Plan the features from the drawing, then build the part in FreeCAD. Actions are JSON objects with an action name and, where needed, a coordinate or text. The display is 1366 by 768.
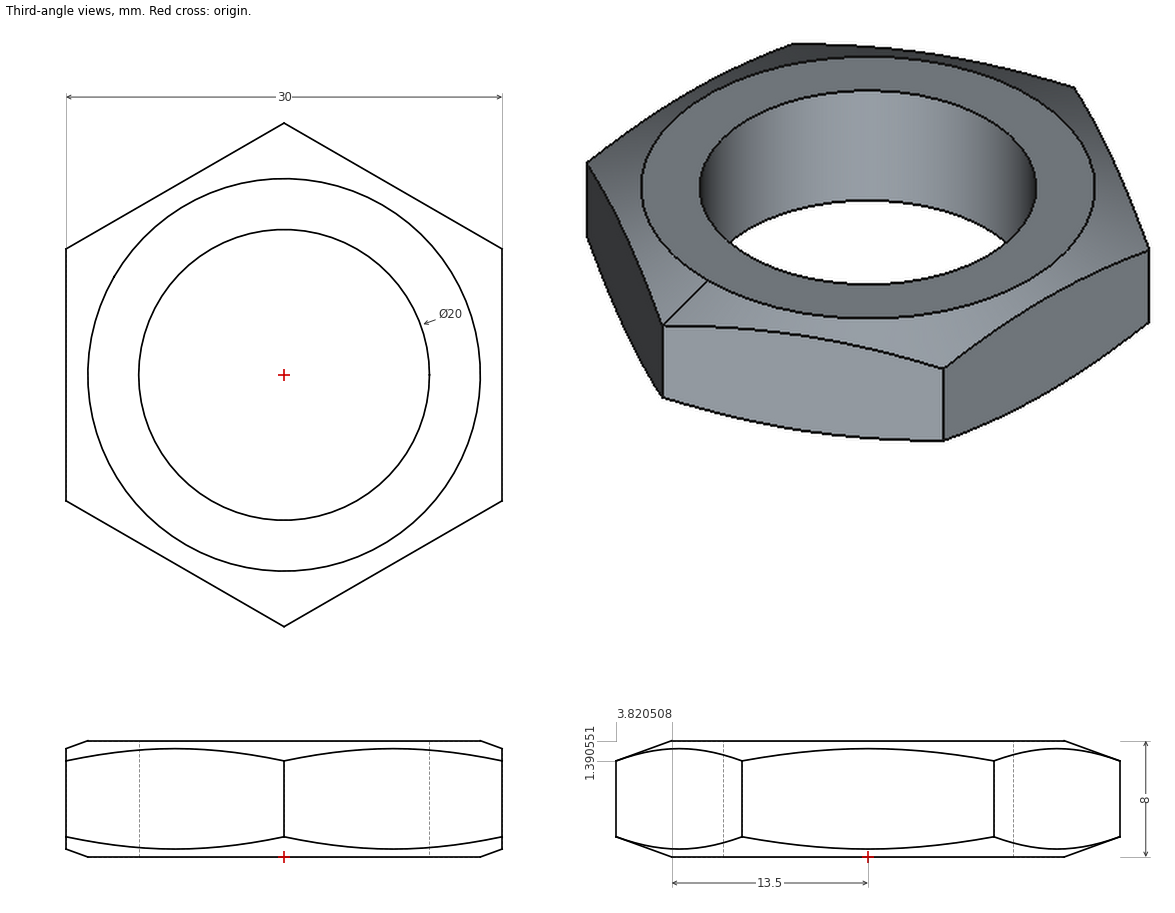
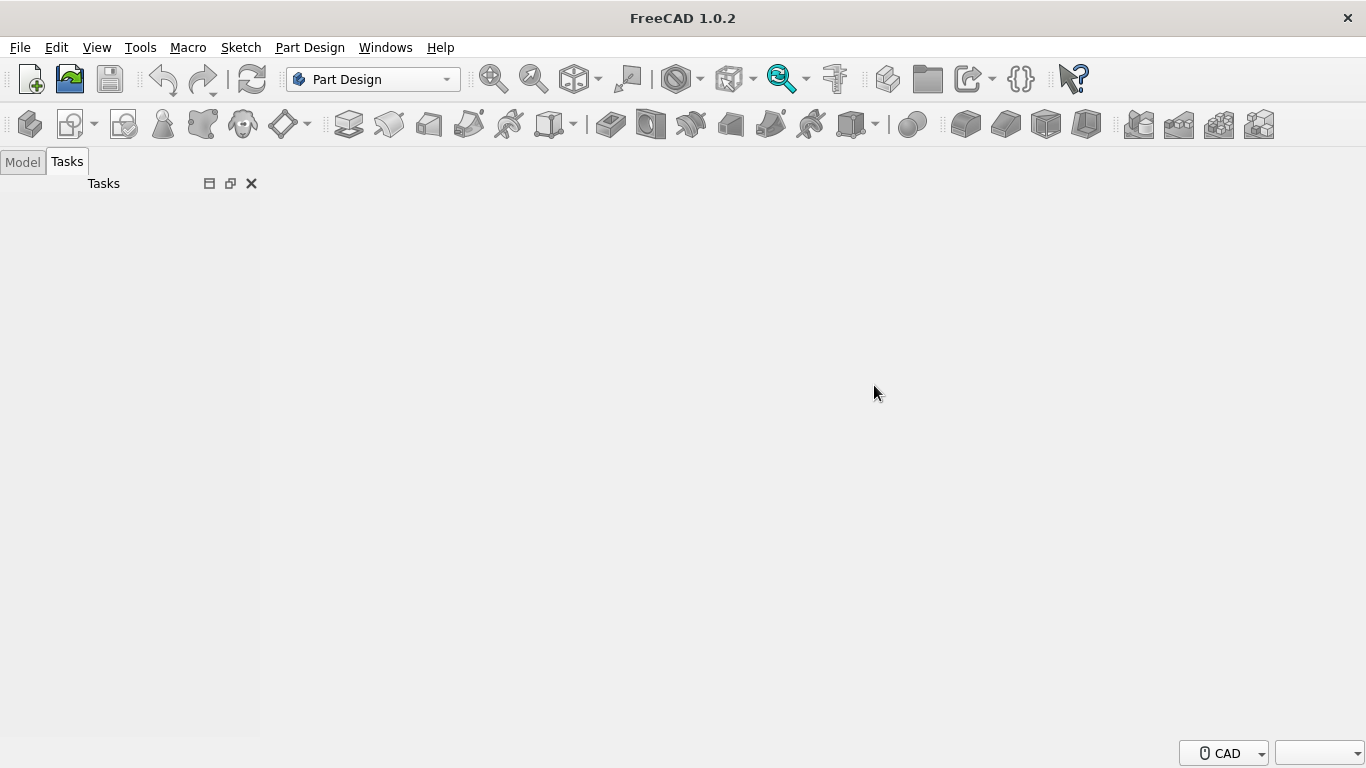
{"action": "left_click", "coordinate": [30, 80]}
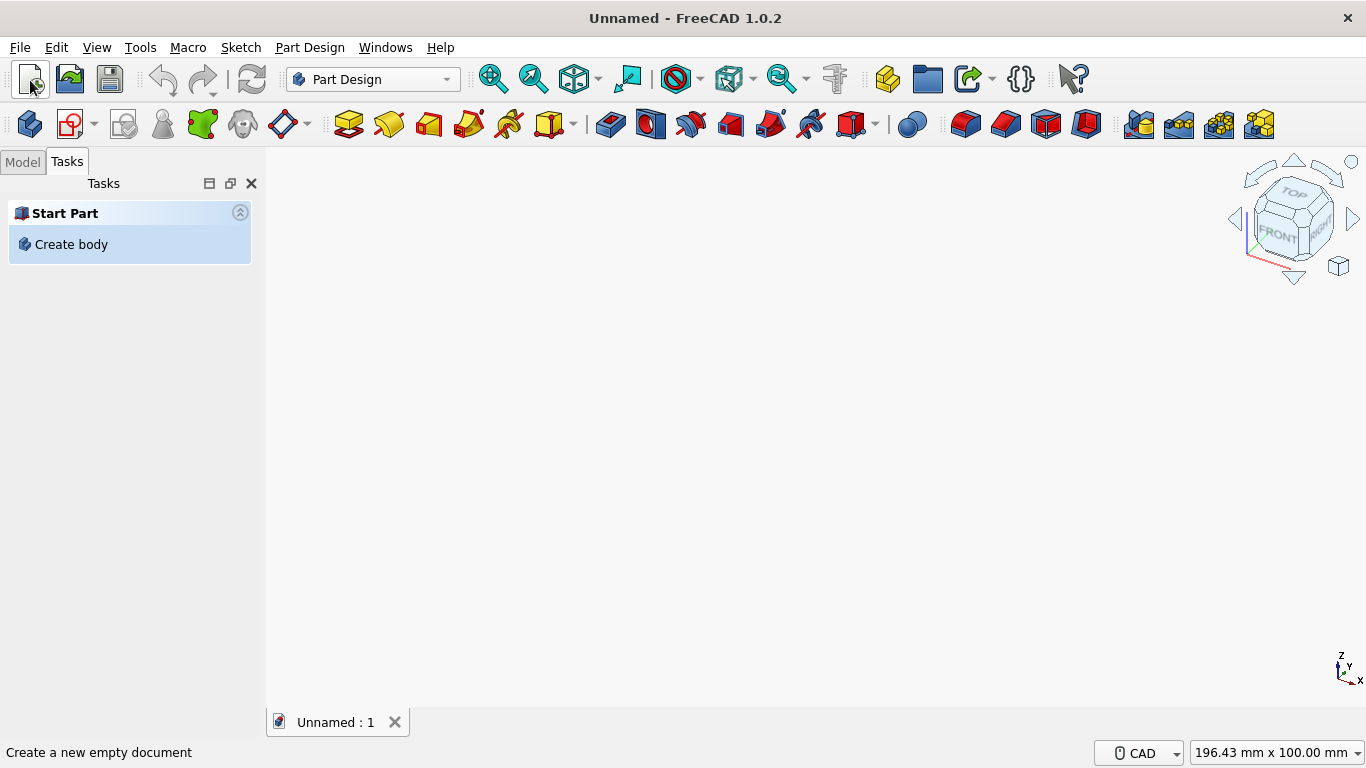
{"action": "left_click", "coordinate": [70, 124]}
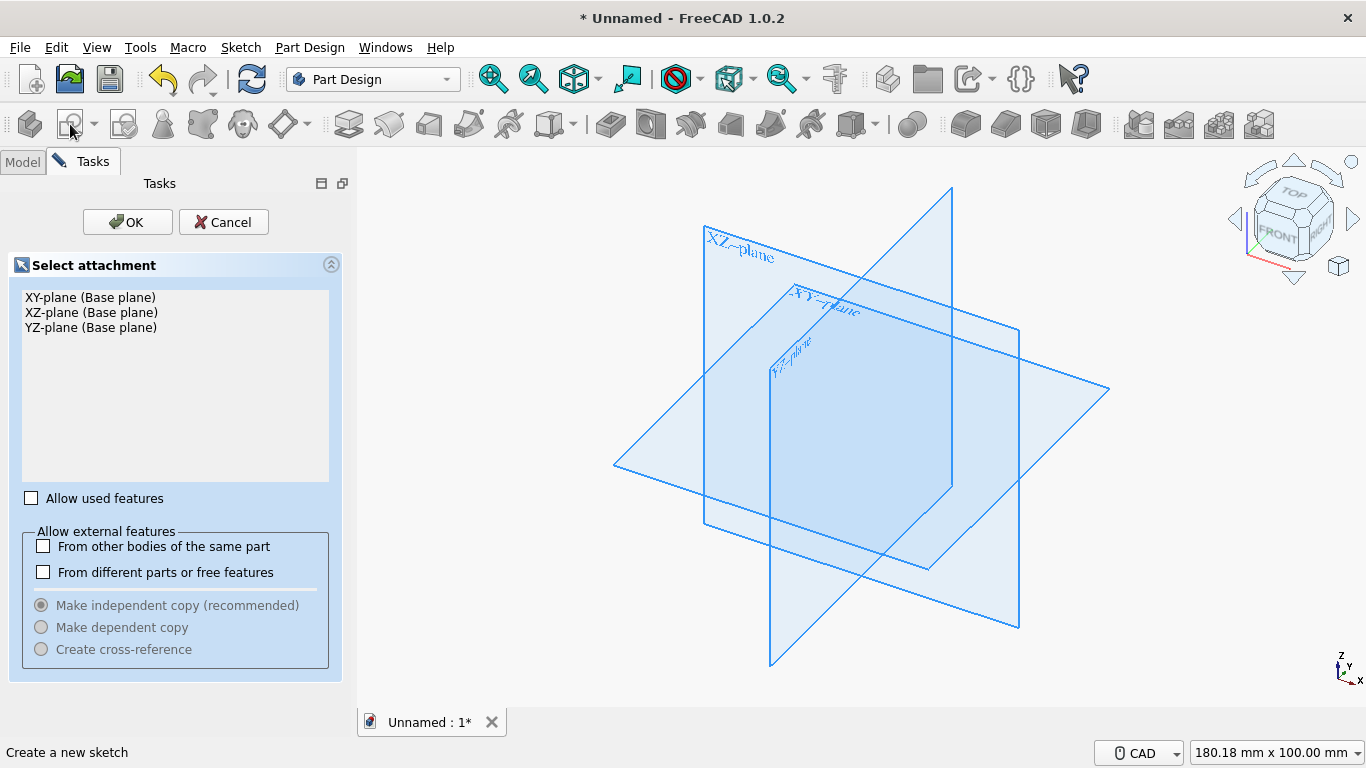
{"action": "left_click", "coordinate": [82, 298]}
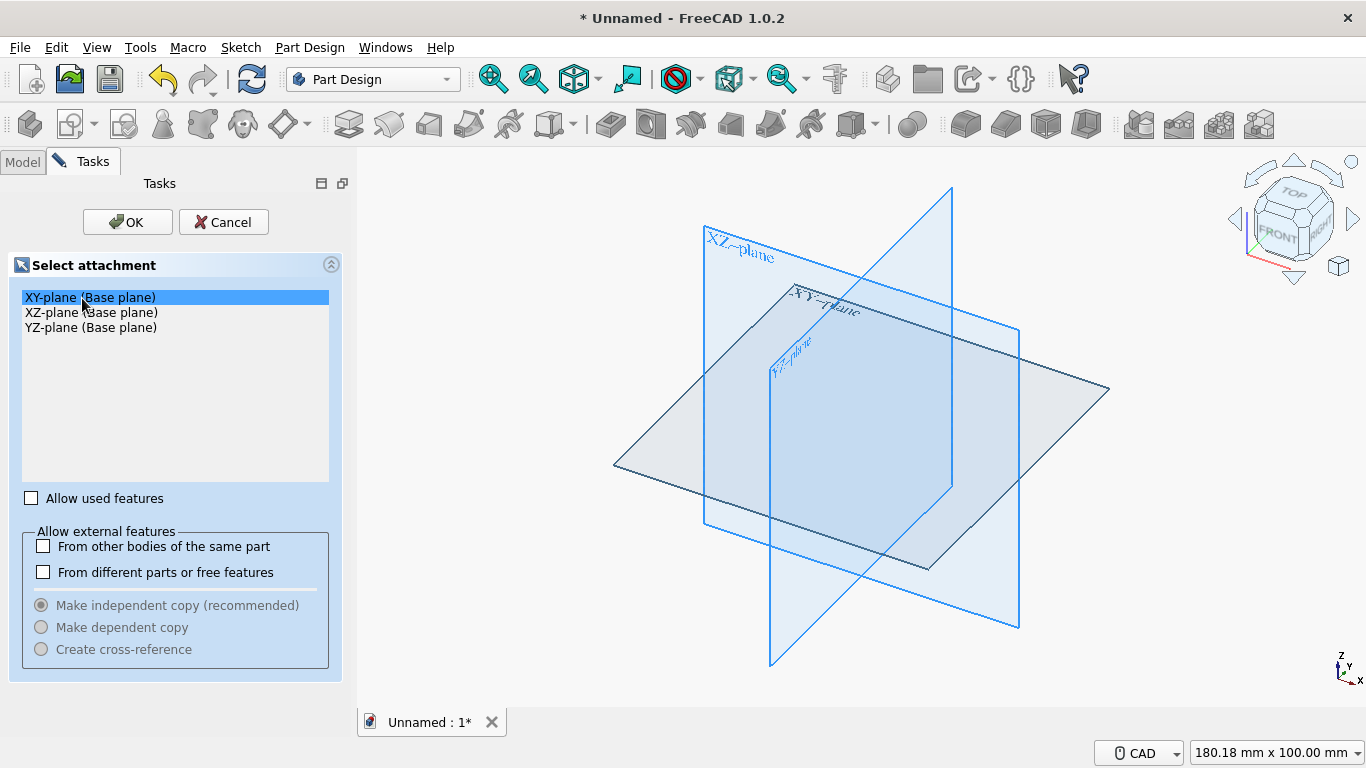
{"action": "left_click", "coordinate": [128, 222]}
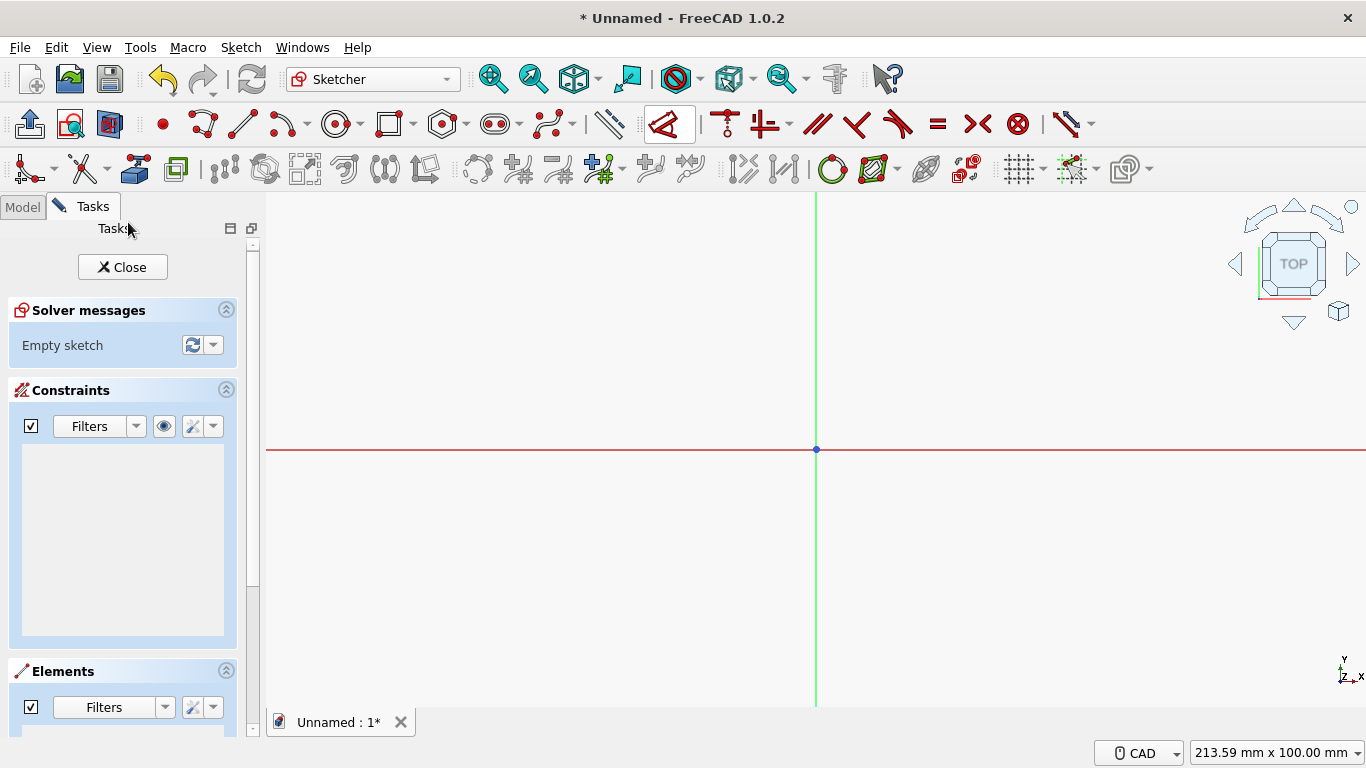
{"action": "scroll", "coordinate": [899, 449], "scroll_direction": "up", "scroll_amount": 3}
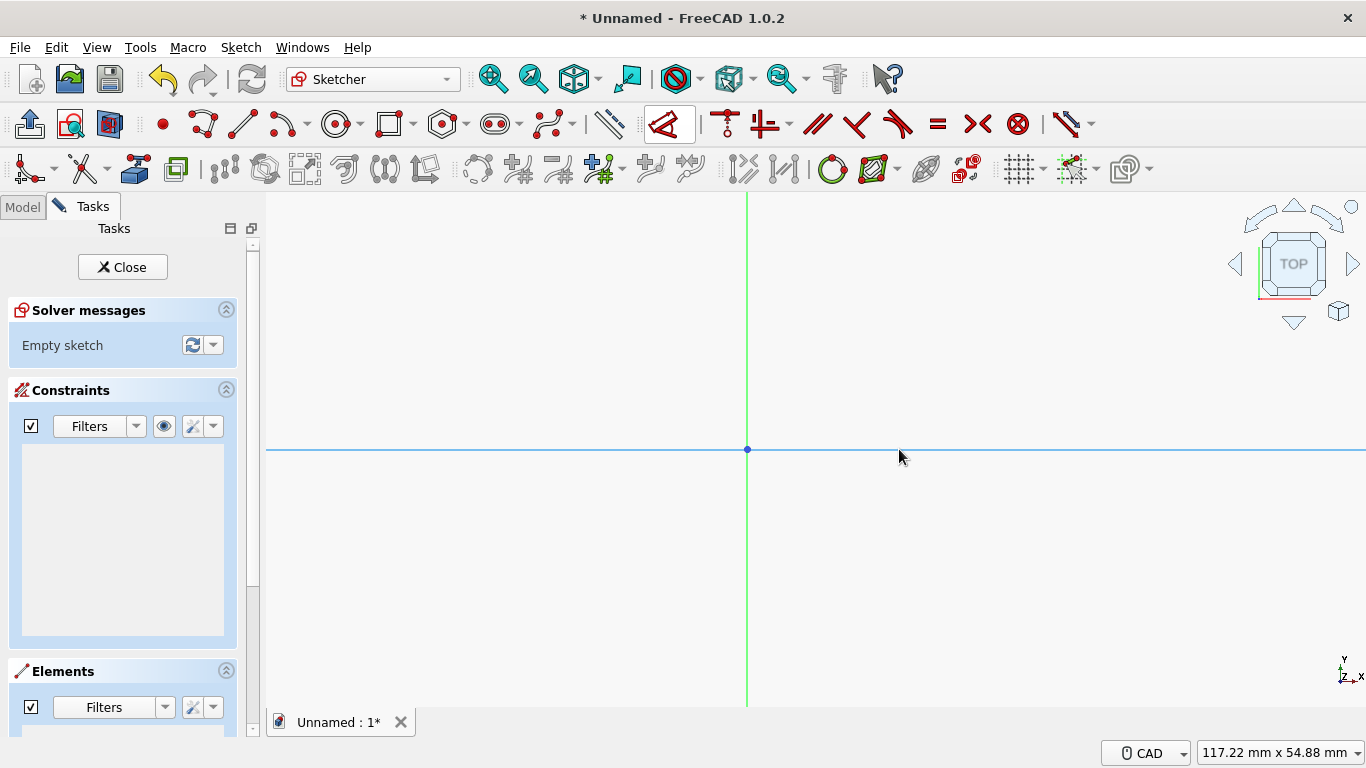
{"action": "left_click", "coordinate": [442, 124]}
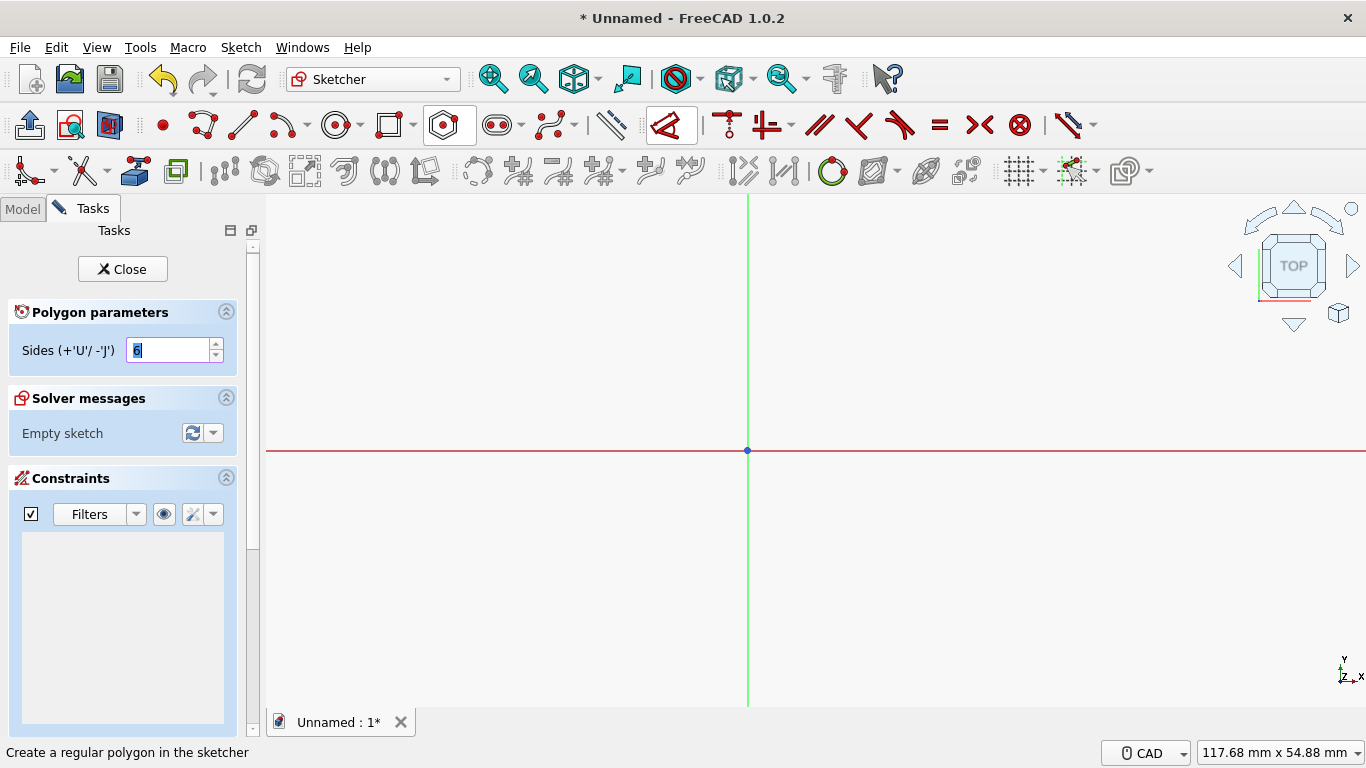
{"action": "left_click", "coordinate": [748, 450]}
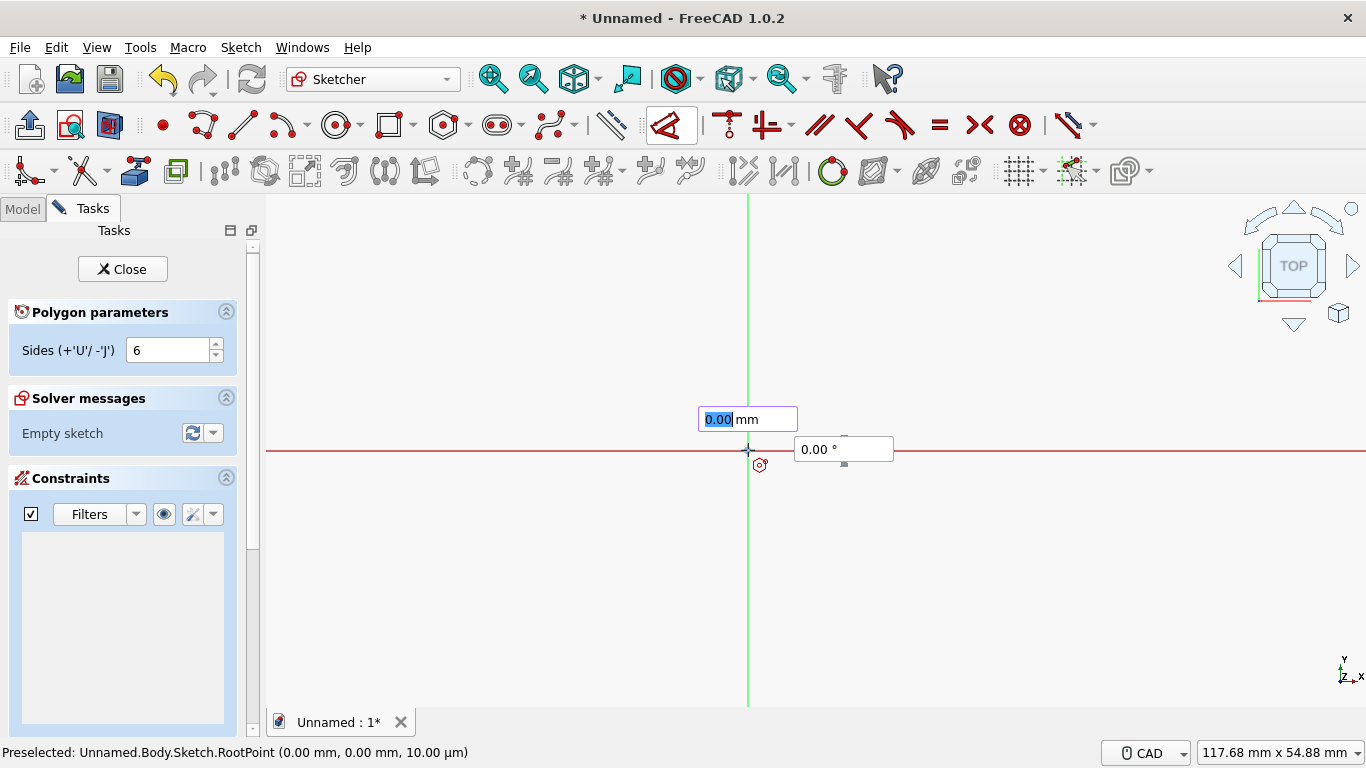
{"action": "left_click", "coordinate": [748, 289]}
{"action": "right_click", "coordinate": [748, 289]}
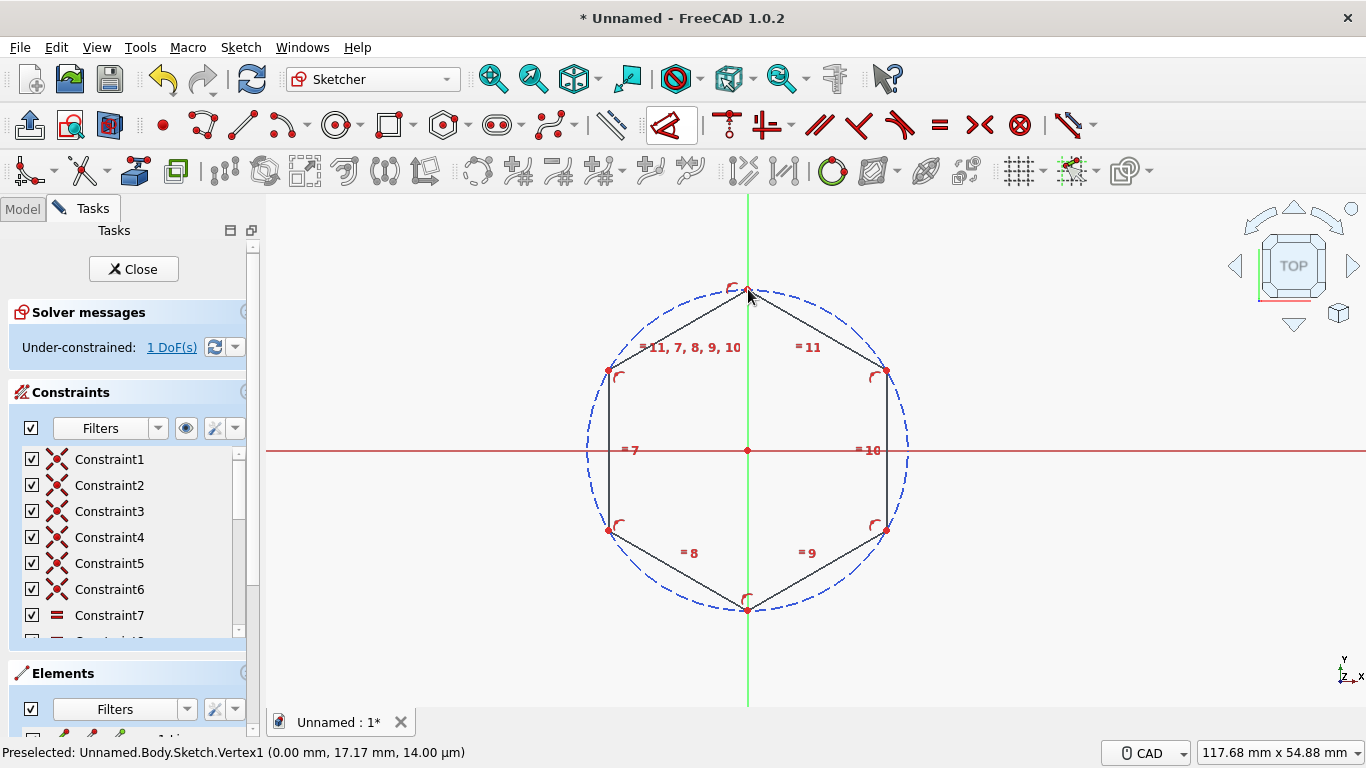
{"action": "key", "text": "d"}